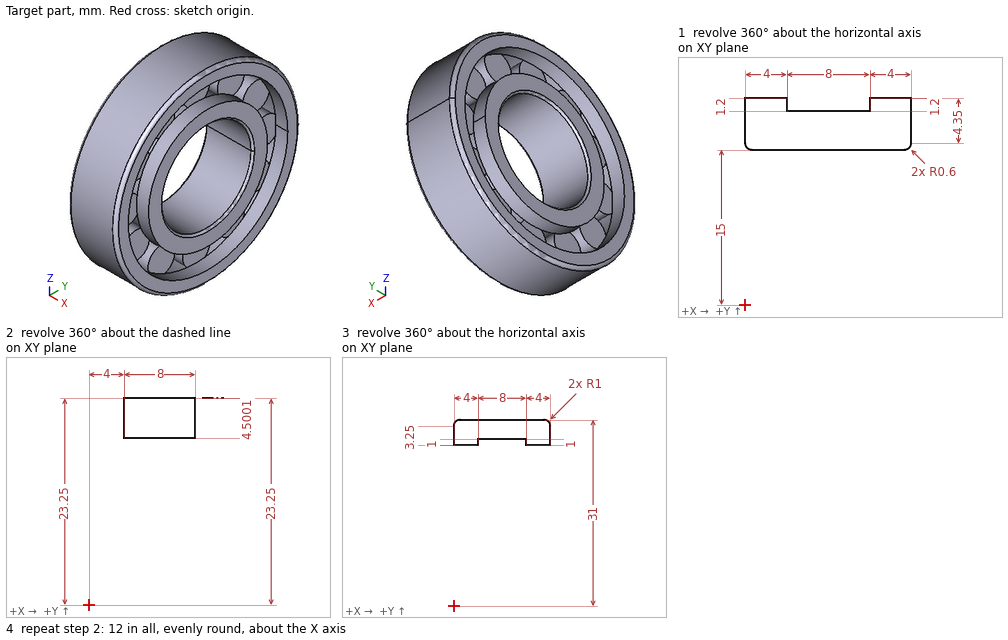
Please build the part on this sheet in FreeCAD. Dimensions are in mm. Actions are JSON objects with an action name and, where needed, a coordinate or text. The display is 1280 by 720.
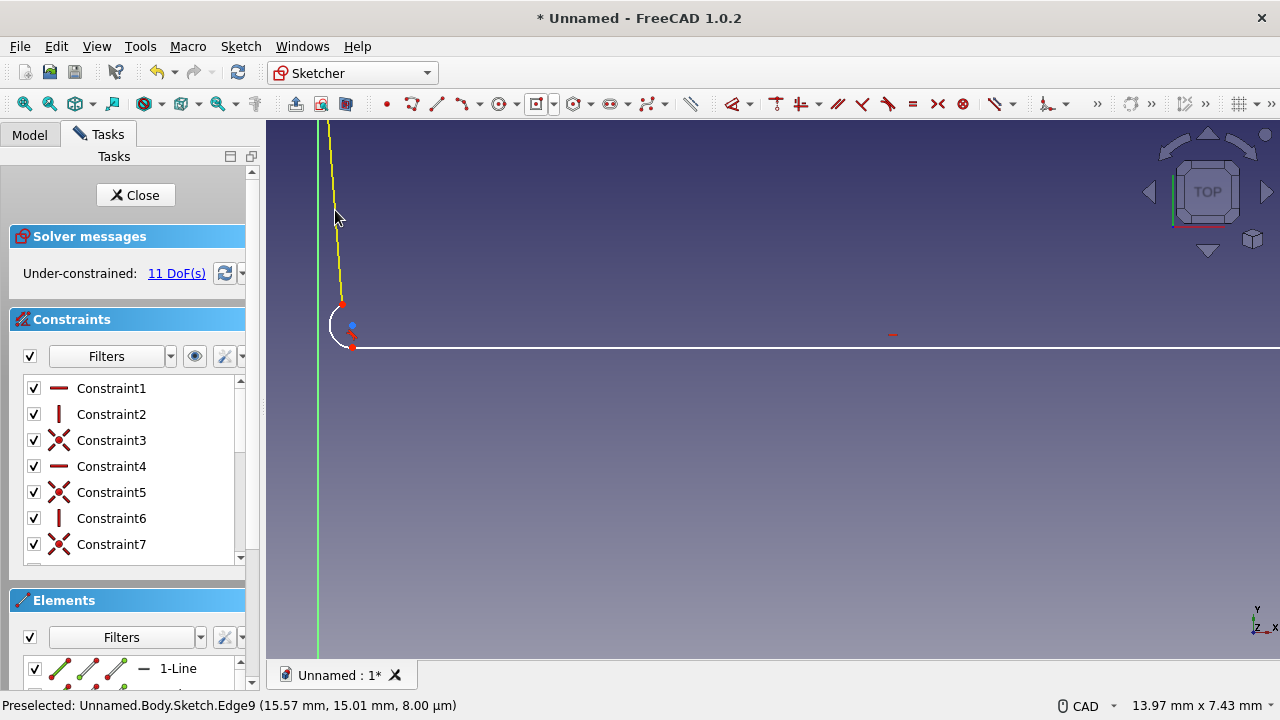
{"action": "left_click", "coordinate": [335, 210]}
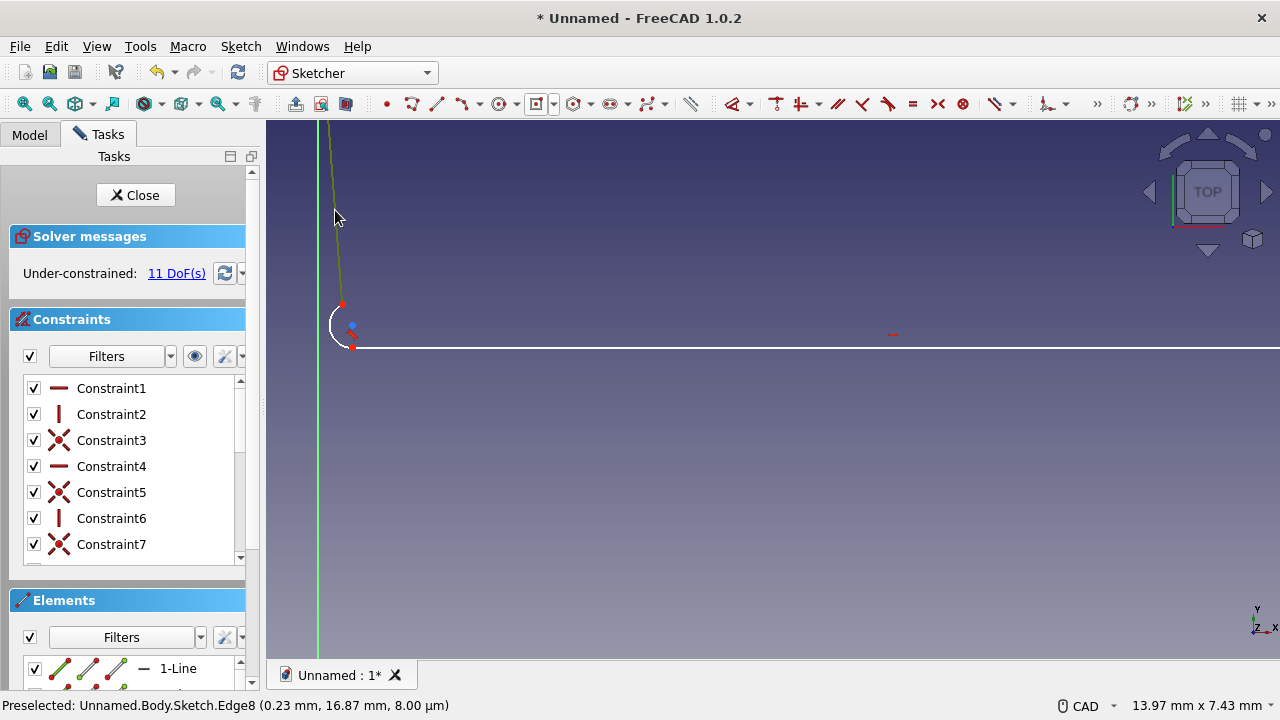
{"action": "left_click", "coordinate": [331, 318]}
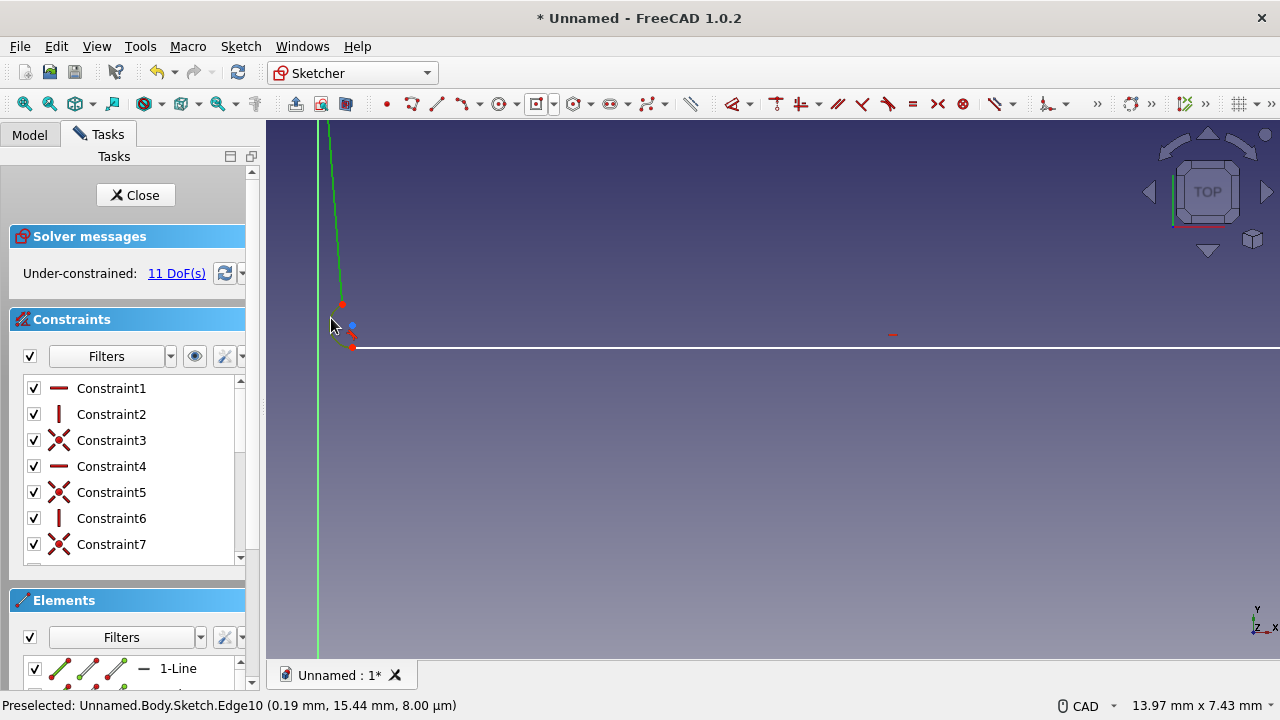
{"action": "key", "text": "t"}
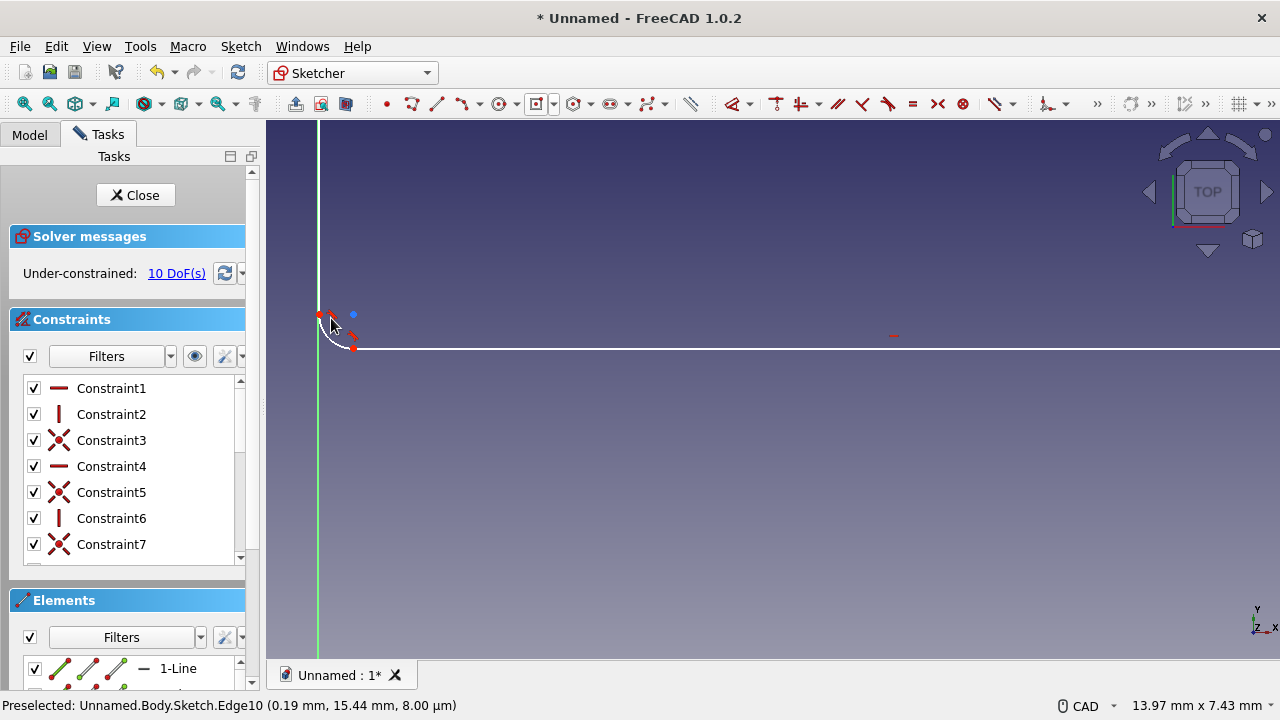
{"action": "scroll", "coordinate": [641, 284], "scroll_direction": "down", "scroll_amount": 7}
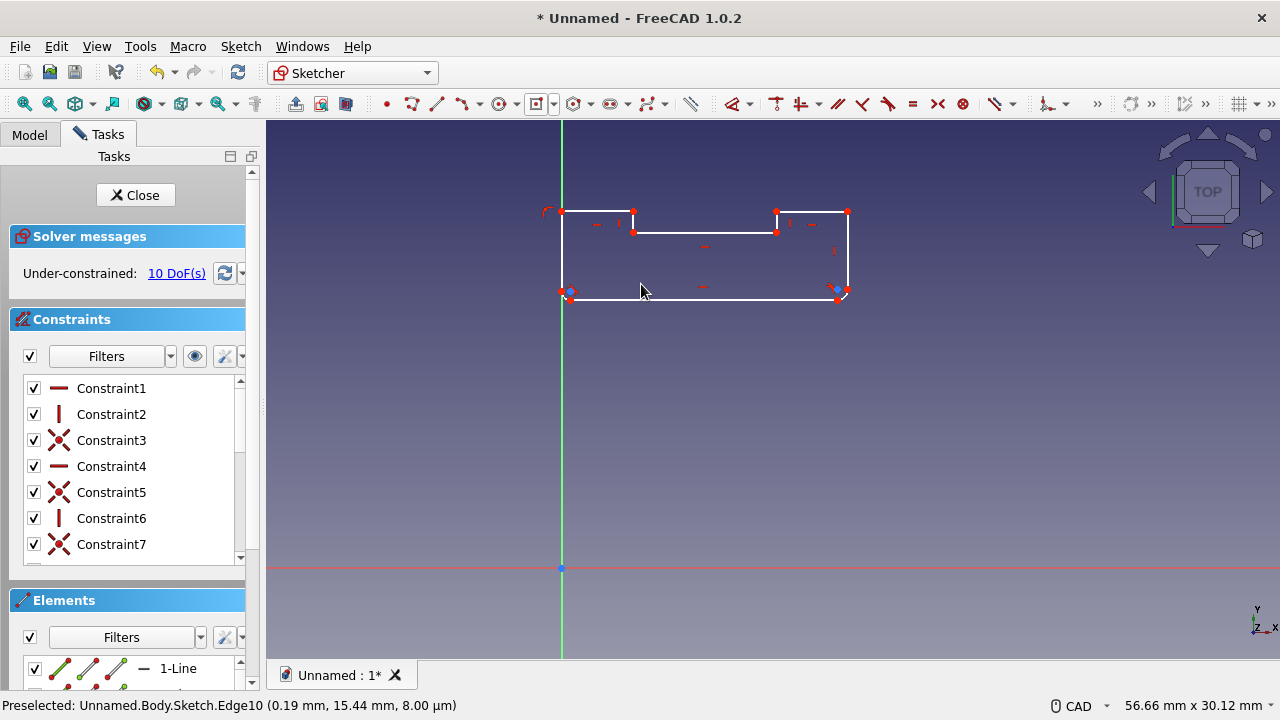
{"action": "left_click", "coordinate": [562, 268]}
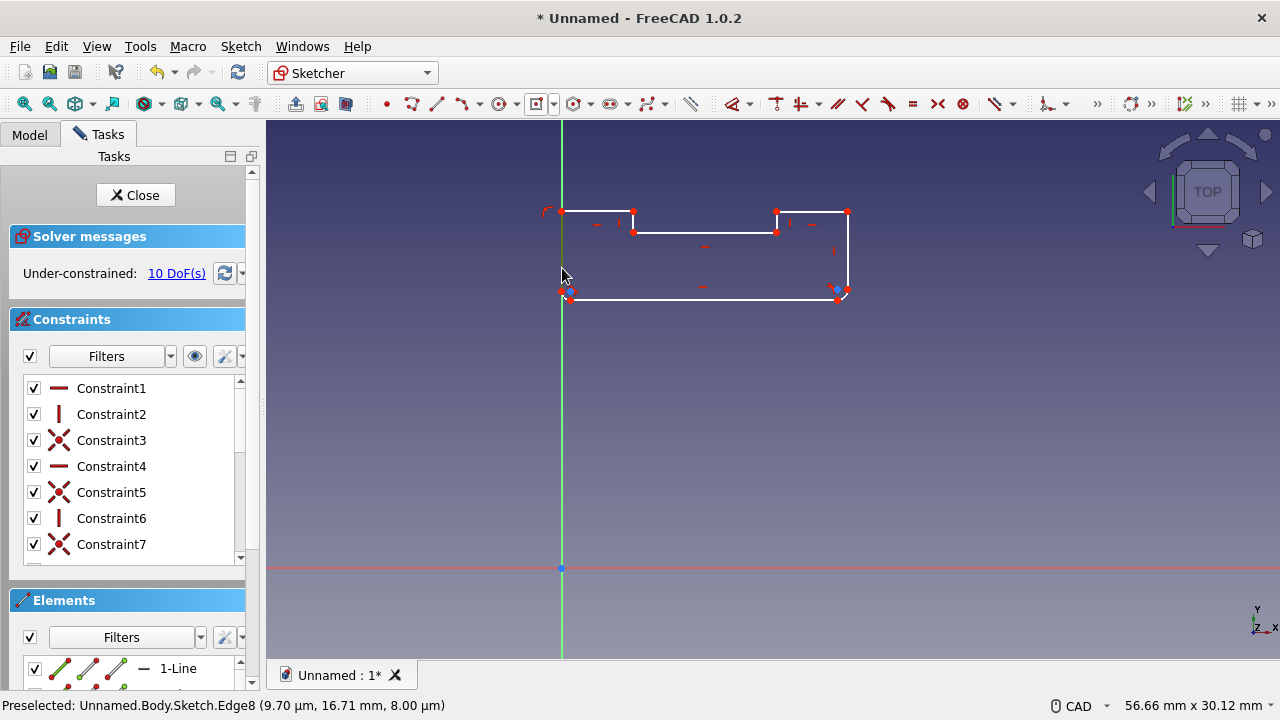
{"action": "key", "text": "v"}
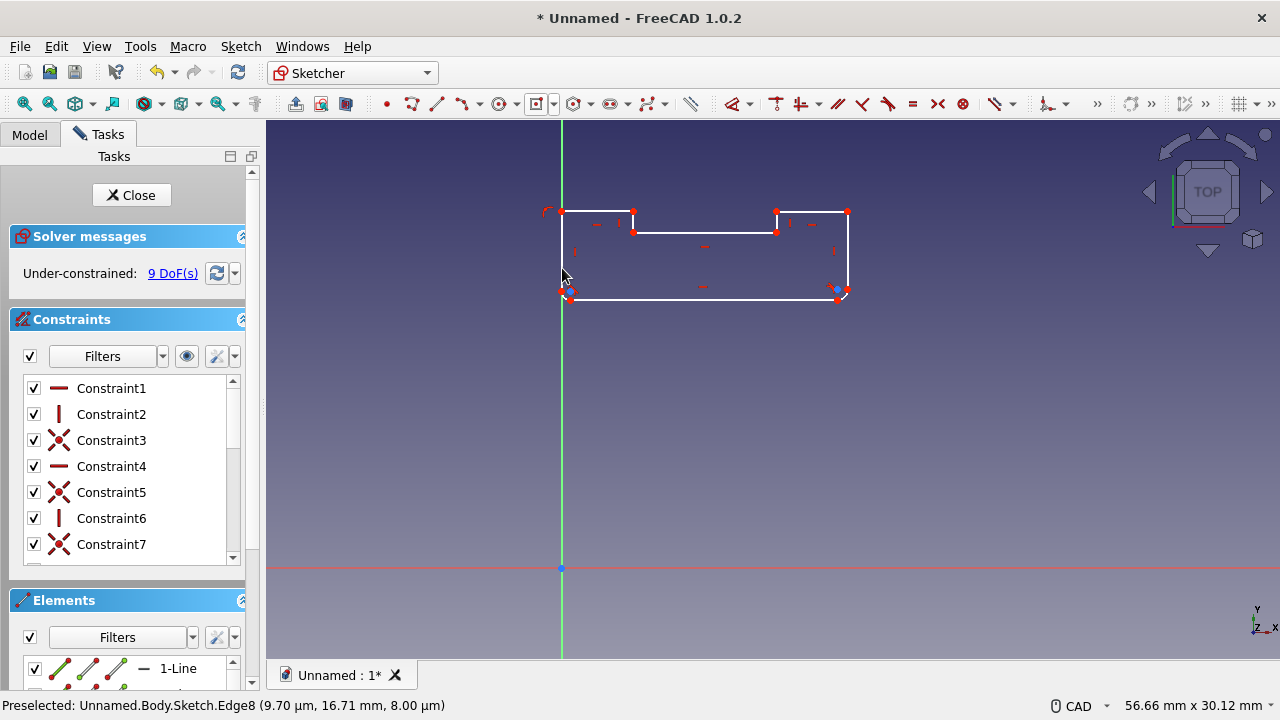
{"action": "scroll", "coordinate": [845, 297], "scroll_direction": "up", "scroll_amount": 3}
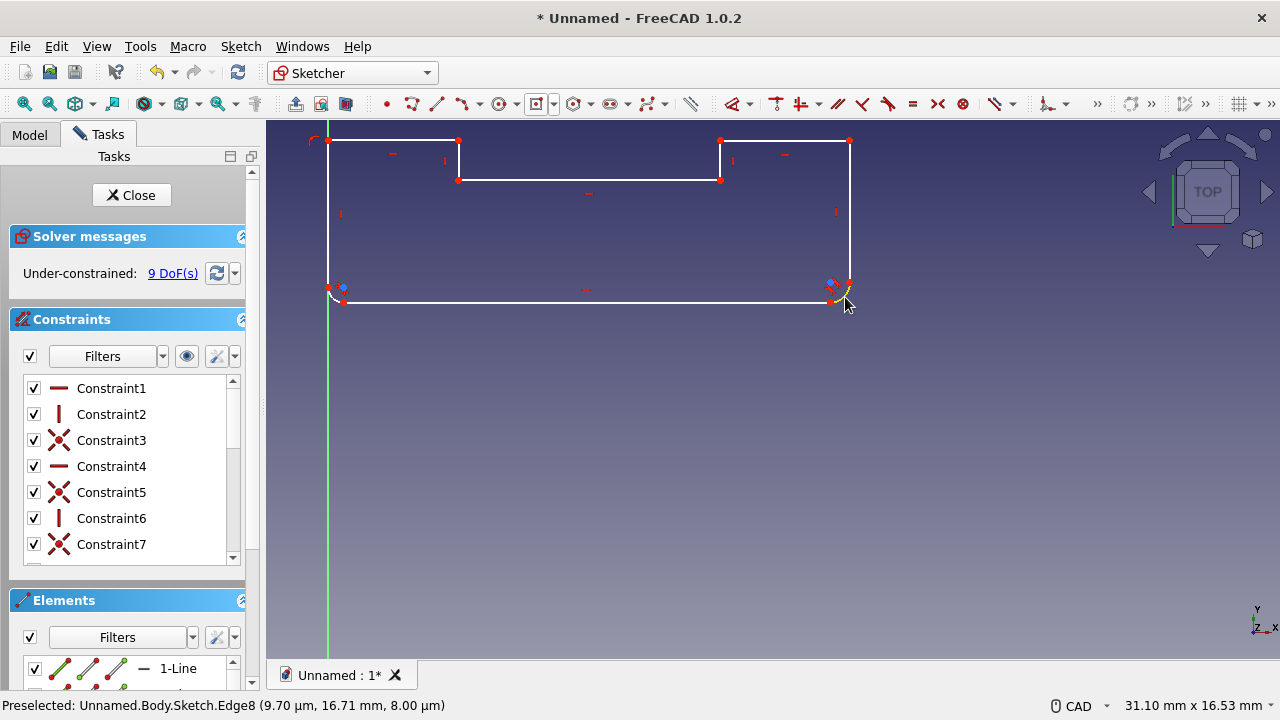
{"action": "left_click", "coordinate": [844, 297]}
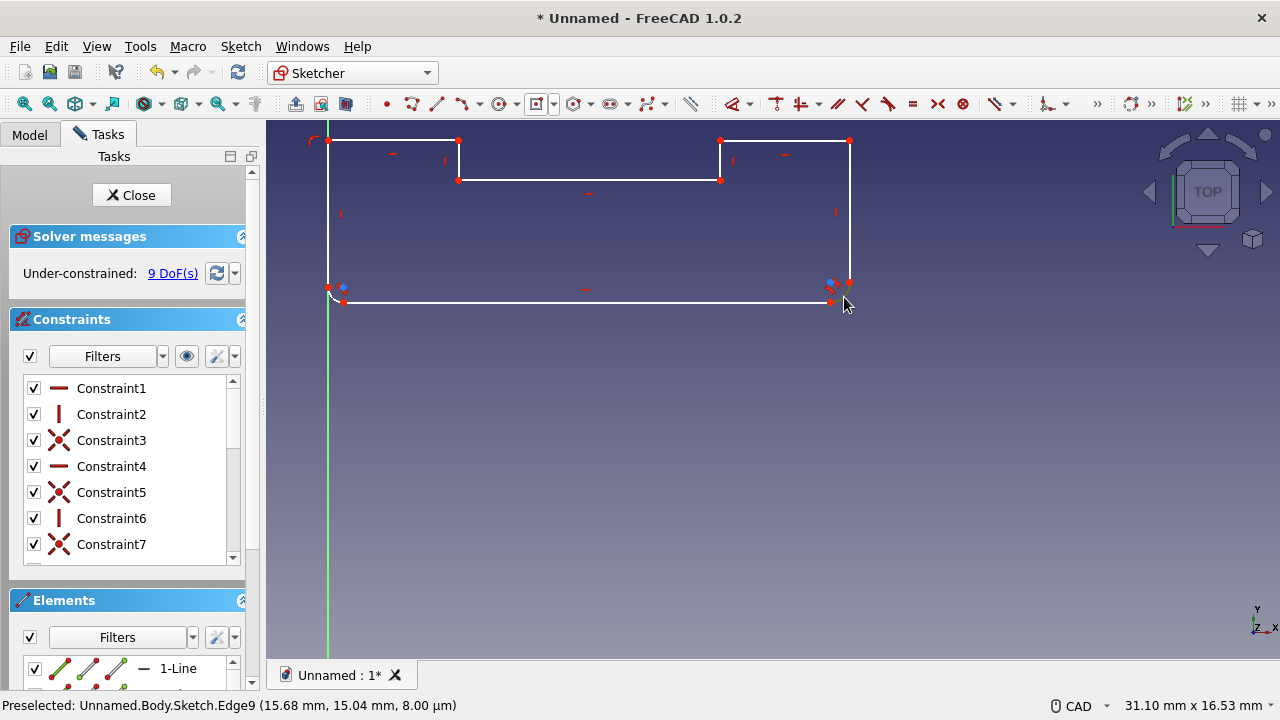
{"action": "scroll", "coordinate": [337, 301], "scroll_direction": "up", "scroll_amount": 4}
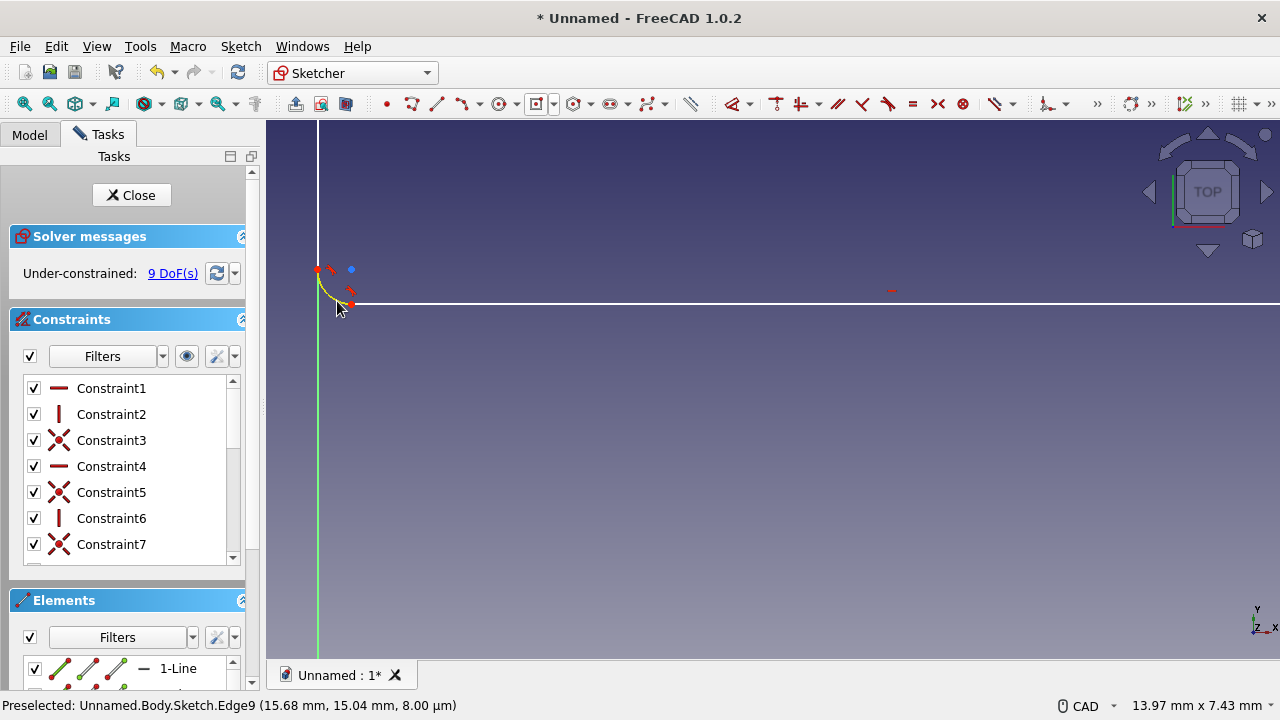
{"action": "left_click", "coordinate": [336, 300]}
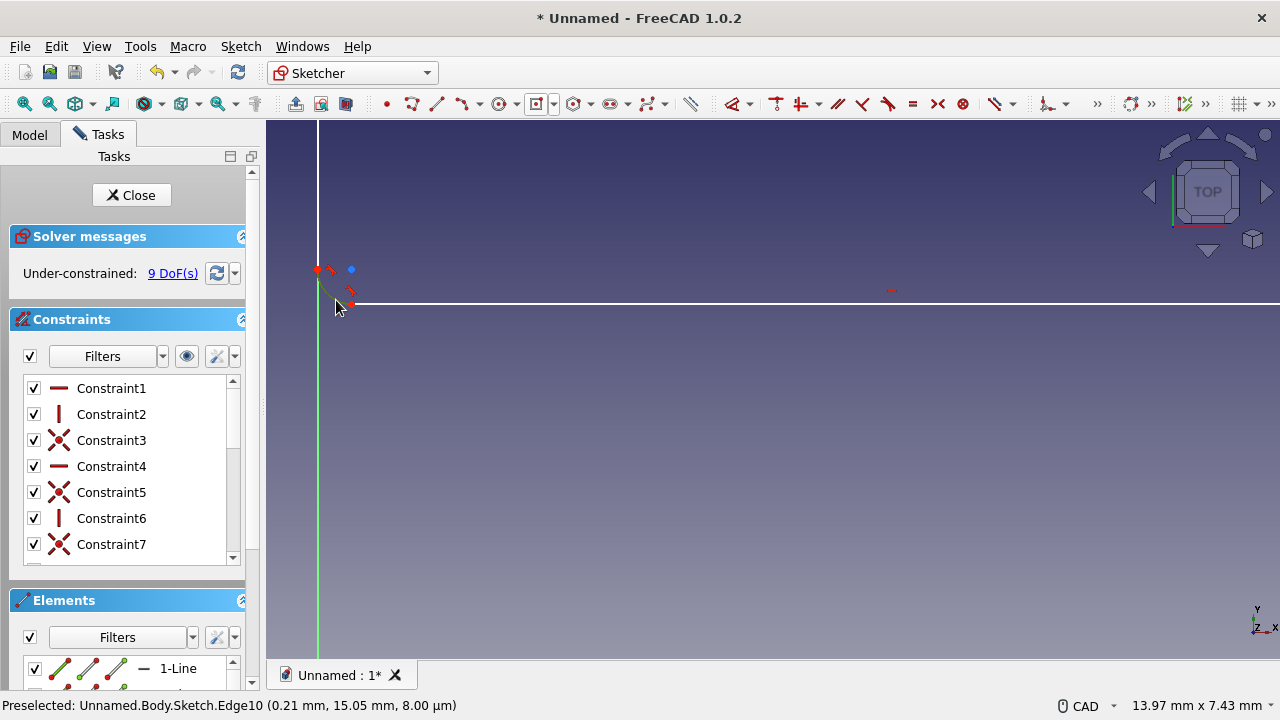
{"action": "left_click", "coordinate": [913, 104]}